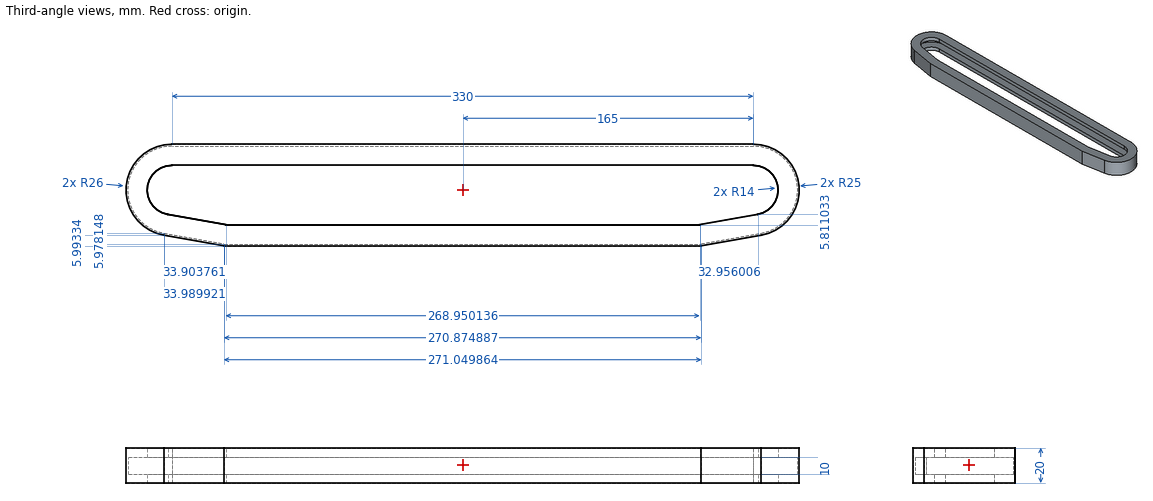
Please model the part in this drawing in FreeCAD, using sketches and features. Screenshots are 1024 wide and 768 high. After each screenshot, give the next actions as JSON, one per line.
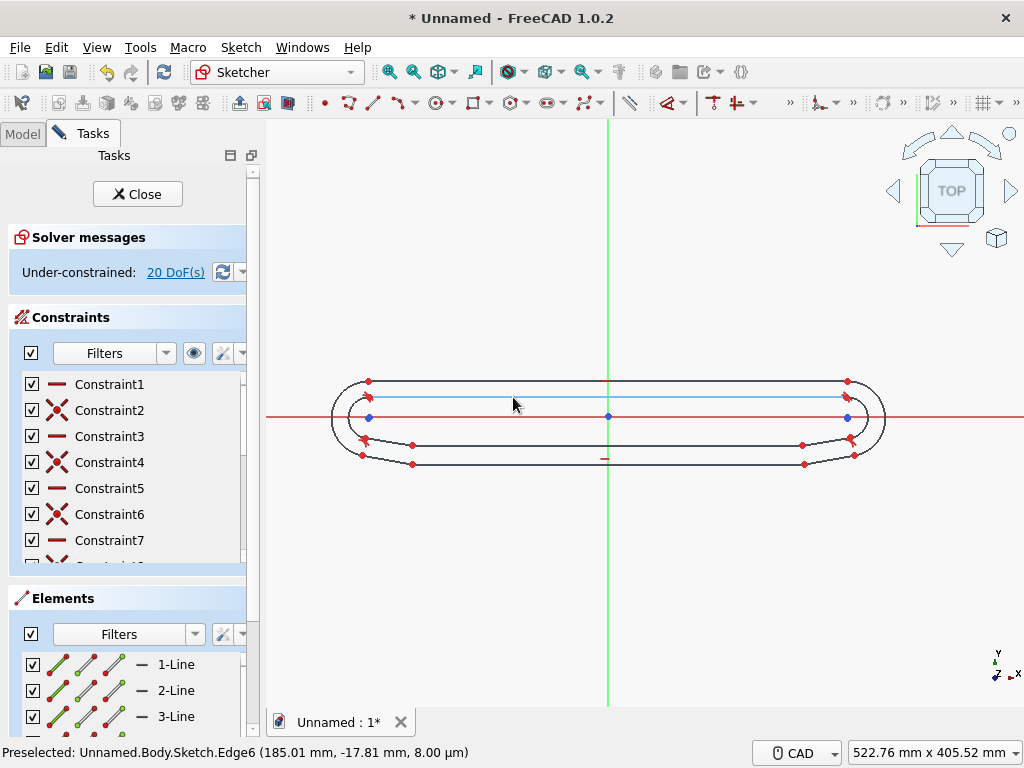
{"action": "left_click", "coordinate": [513, 397]}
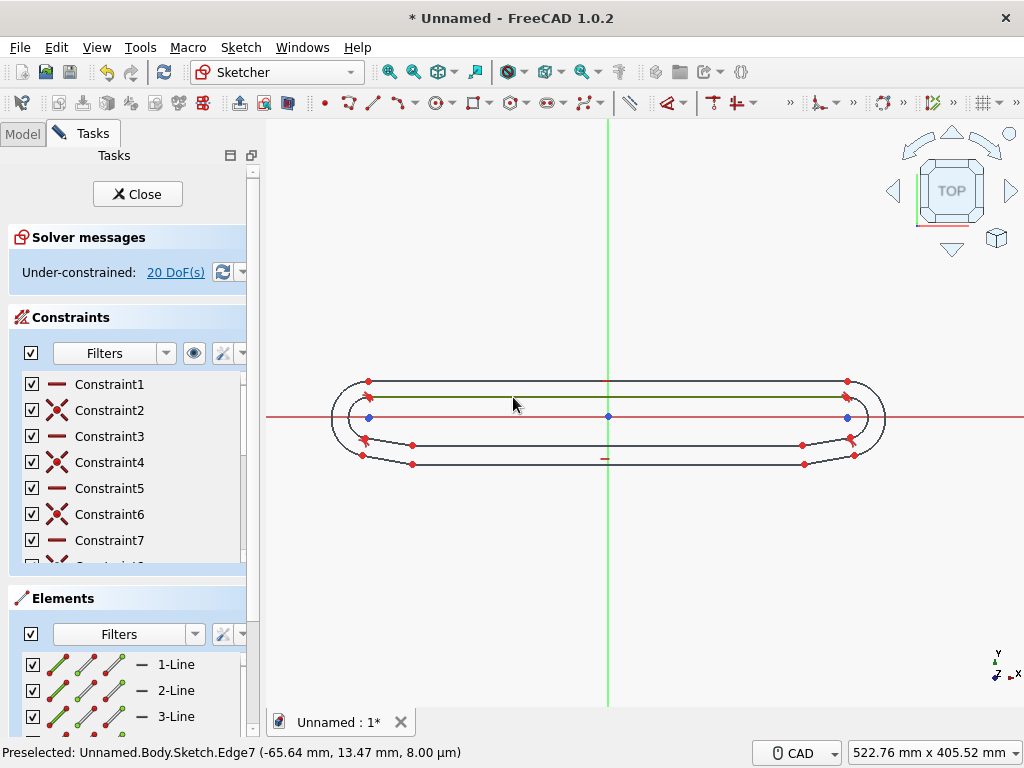
{"action": "left_click", "coordinate": [859, 401]}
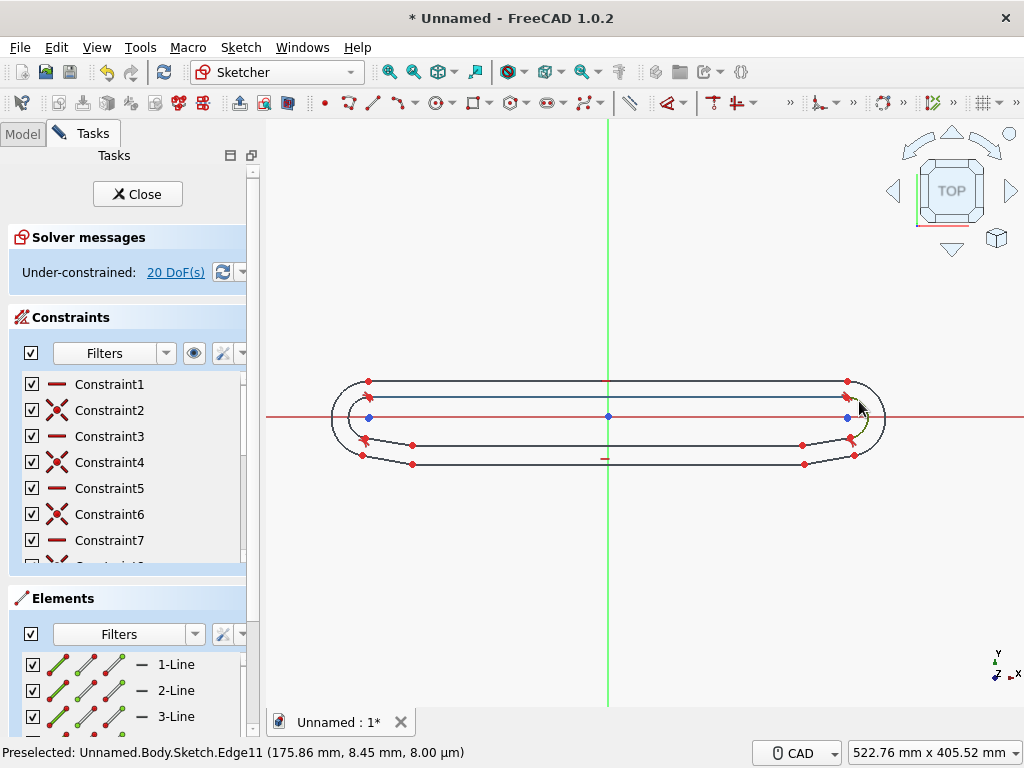
{"action": "key", "text": "t"}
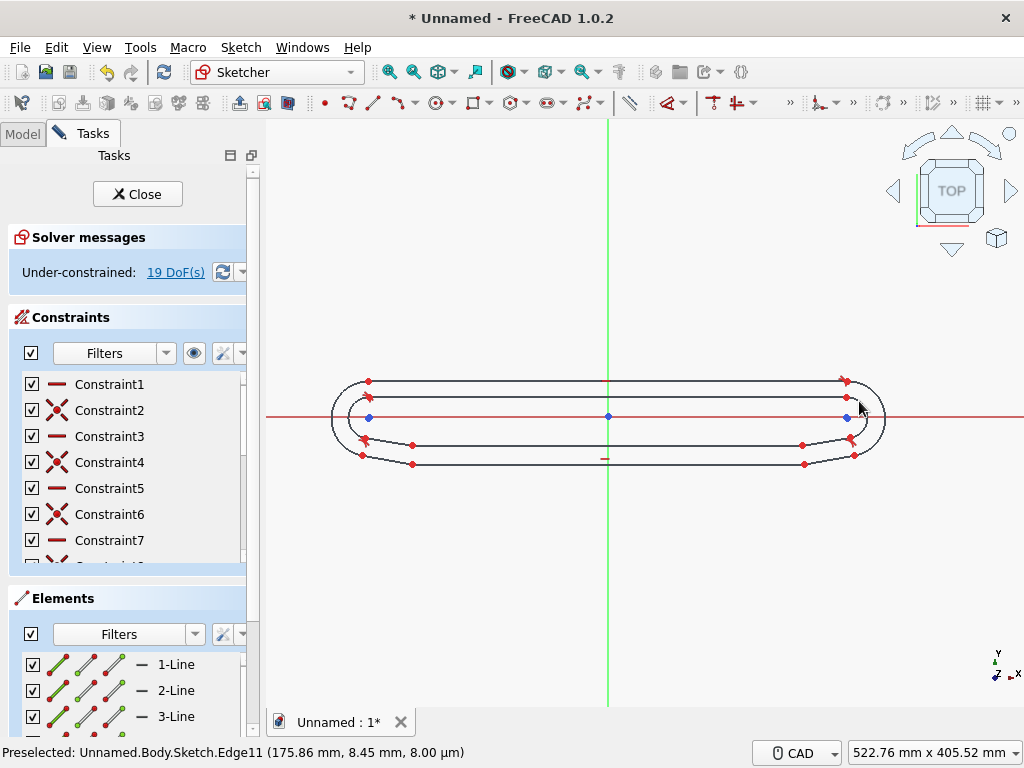
{"action": "left_click", "coordinate": [513, 397]}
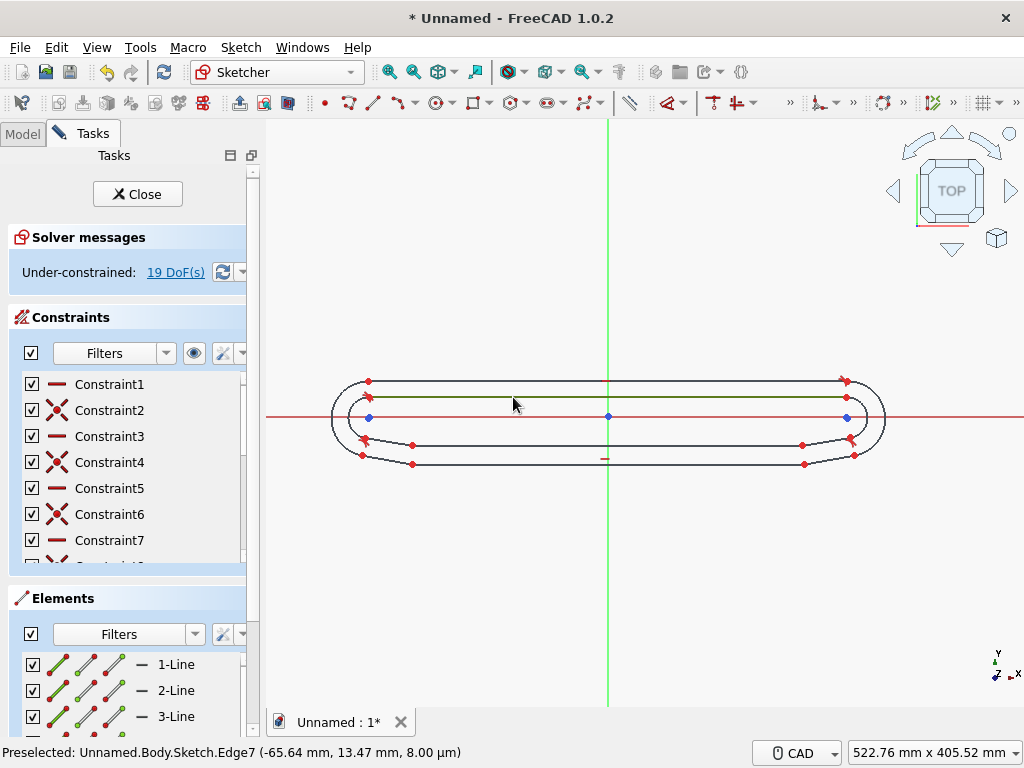
{"action": "left_click", "coordinate": [353, 405]}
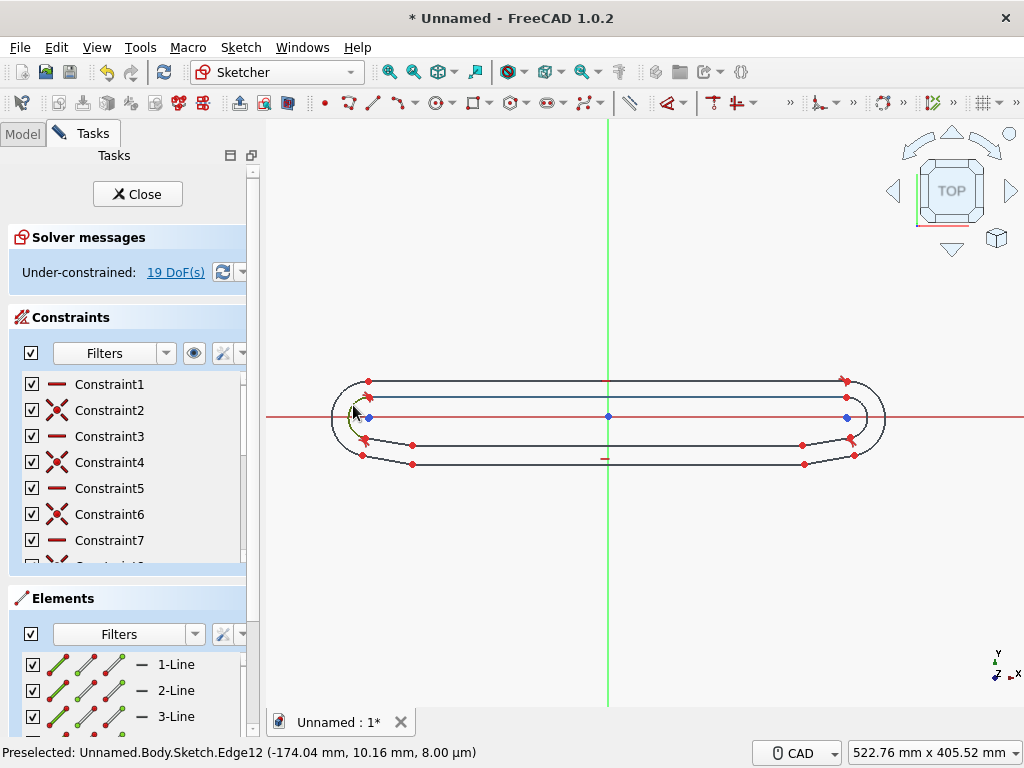
{"action": "key", "text": "t"}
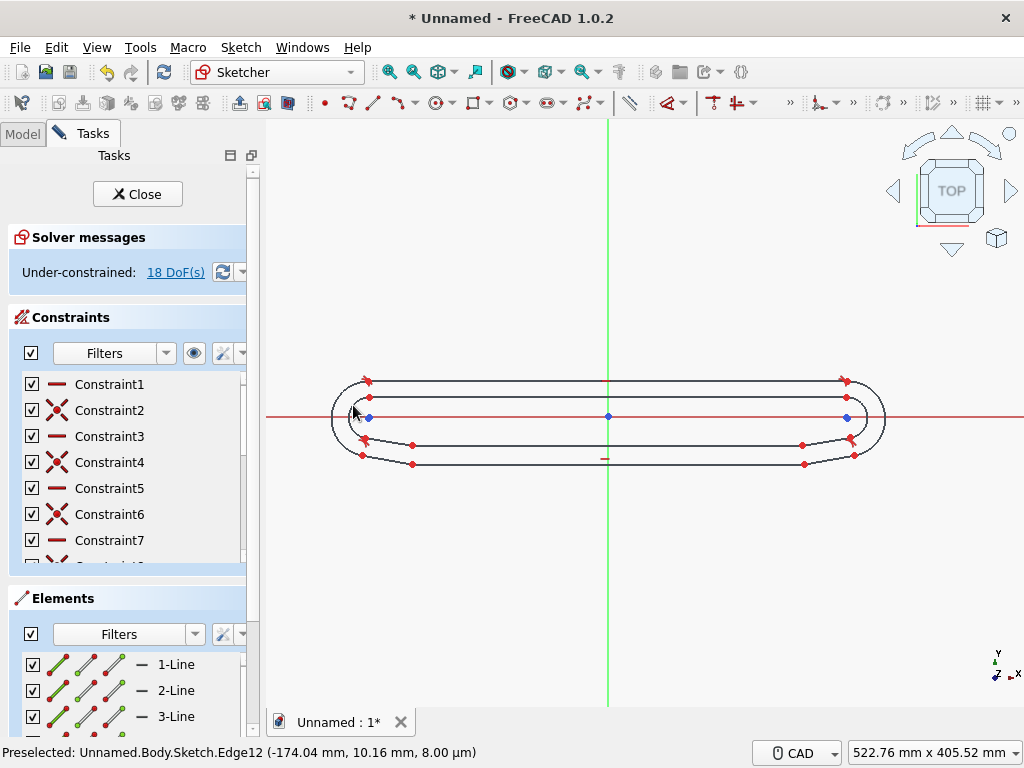
{"action": "left_click", "coordinate": [837, 440]}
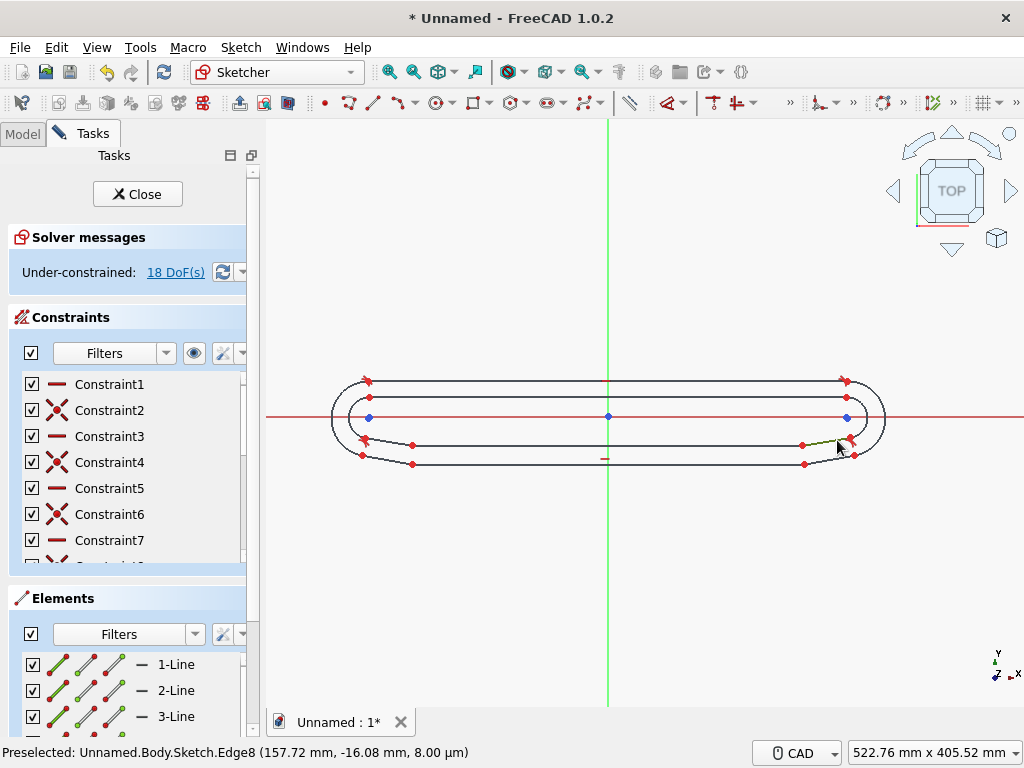
{"action": "left_click", "coordinate": [858, 401]}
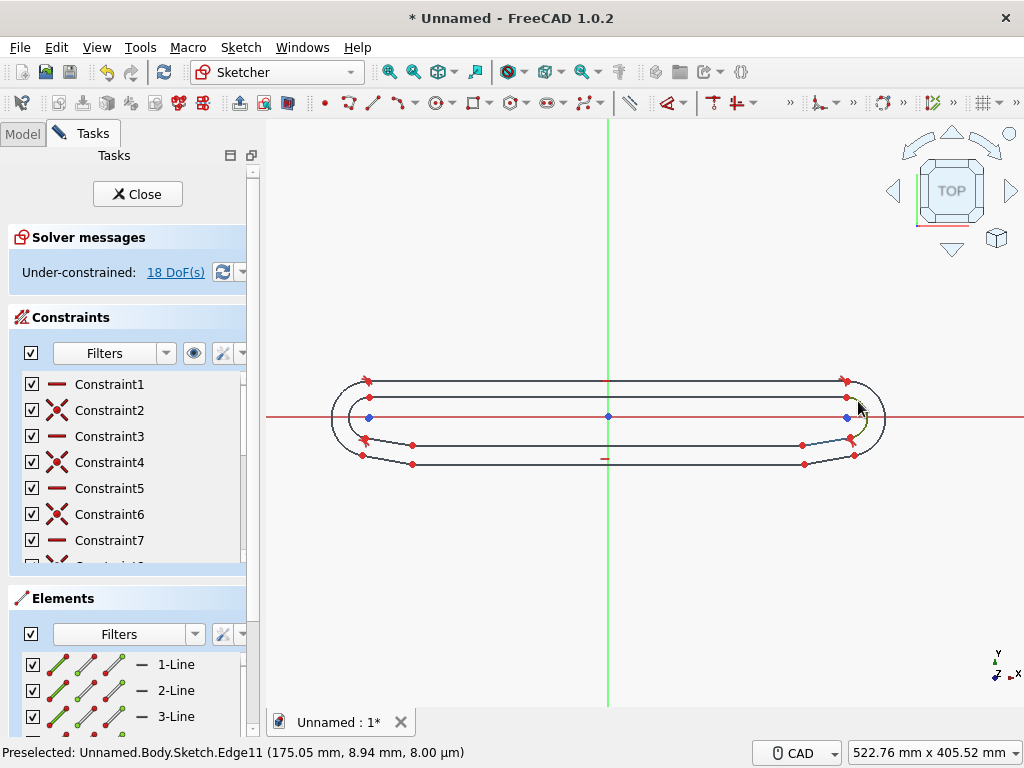
{"action": "key", "text": "t"}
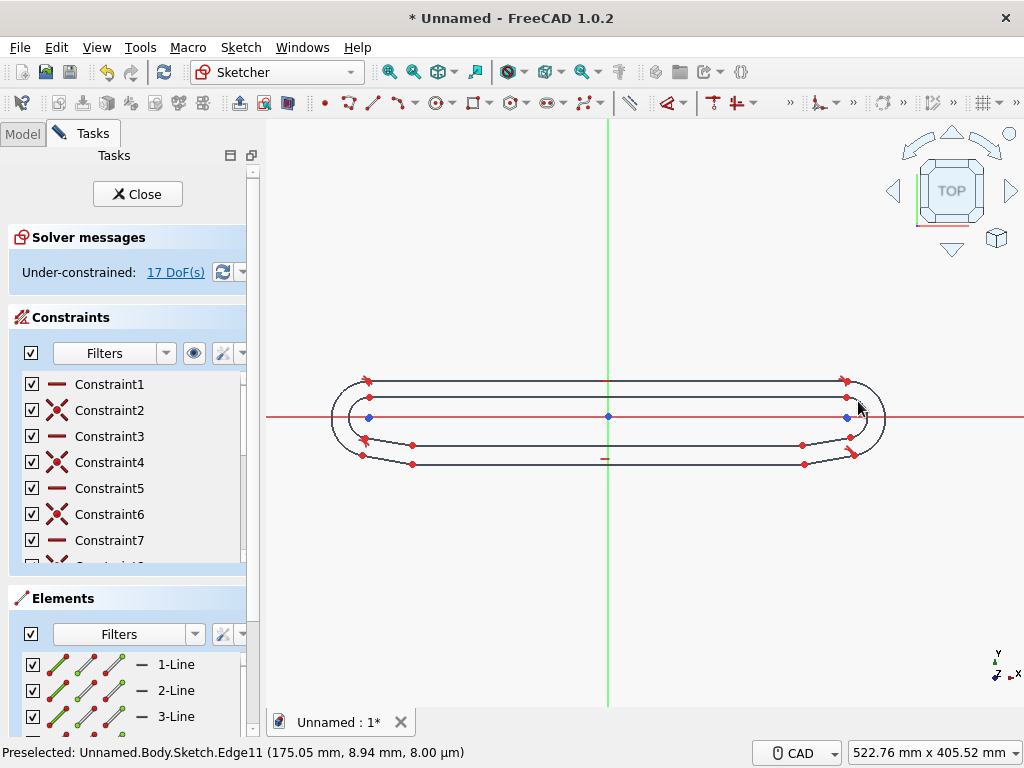
{"action": "left_click", "coordinate": [399, 444]}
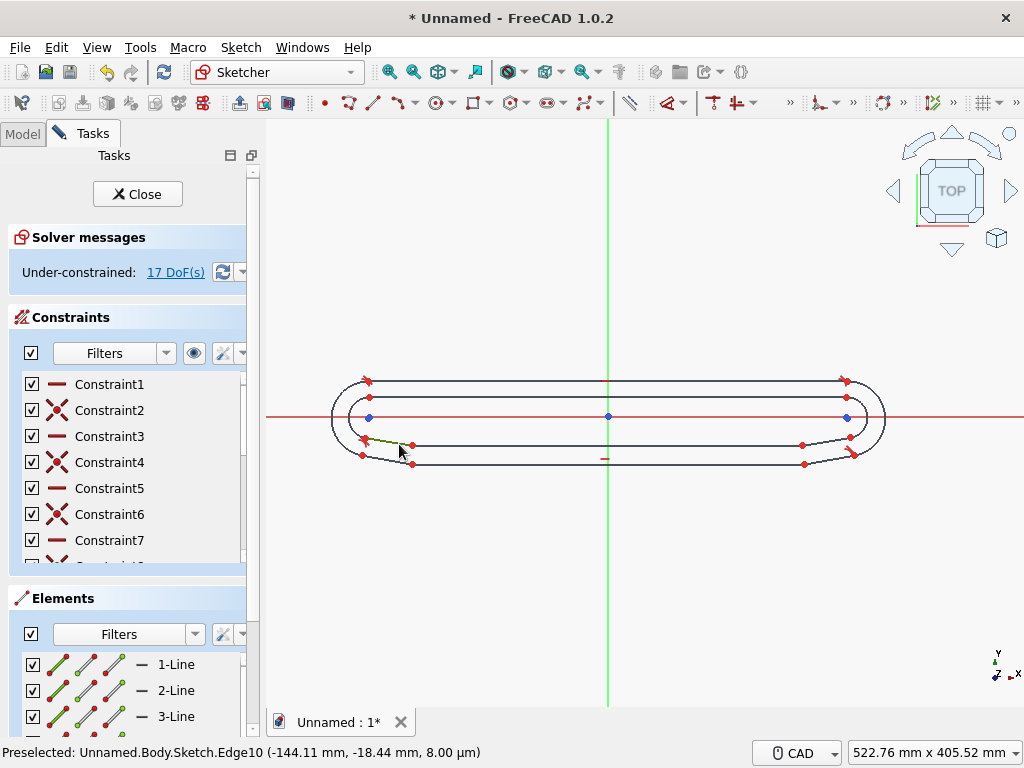
{"action": "left_click", "coordinate": [353, 405]}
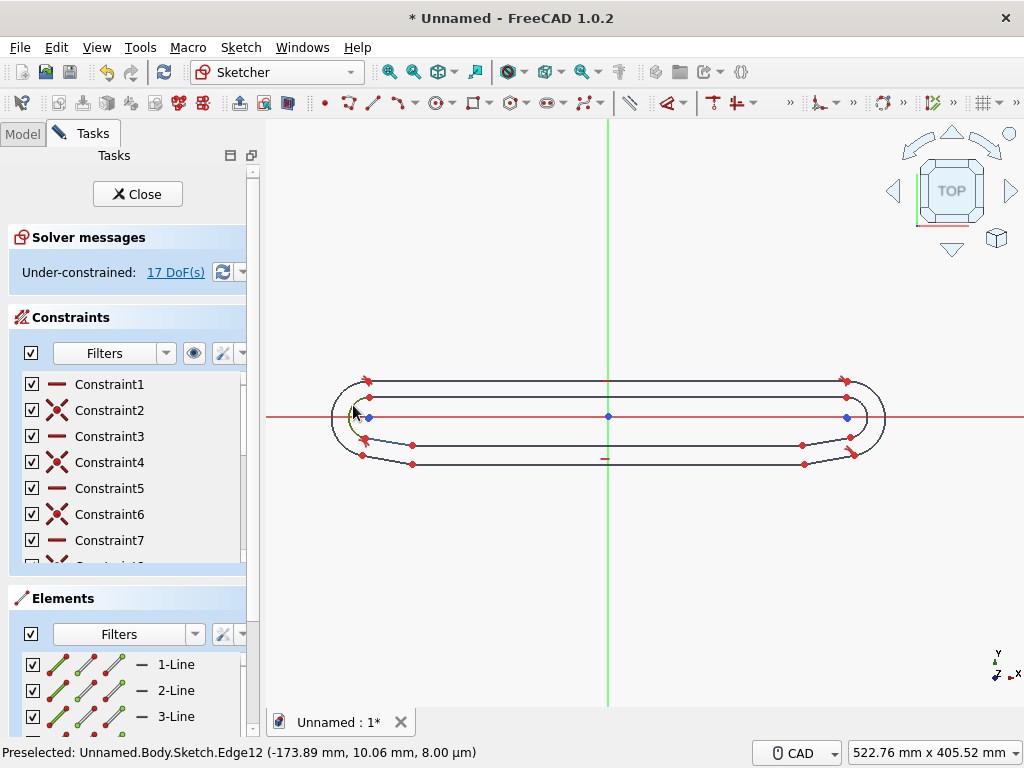
{"action": "key", "text": "t"}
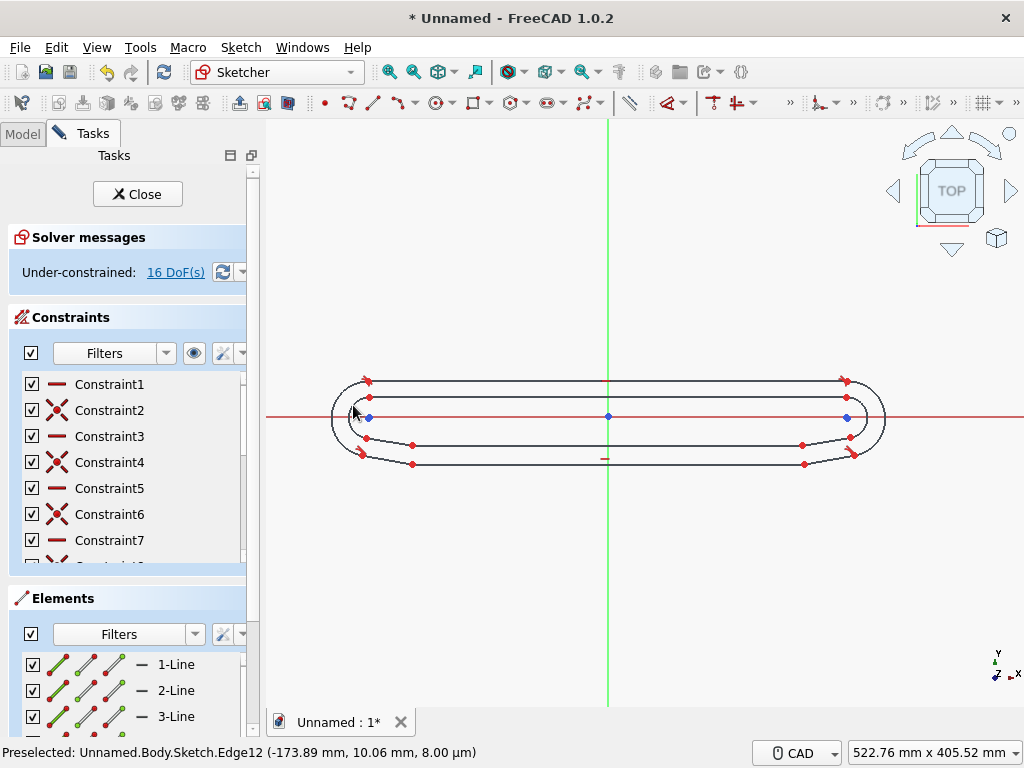
{"action": "scroll", "coordinate": [512, 397], "scroll_direction": "down", "scroll_amount": 2}